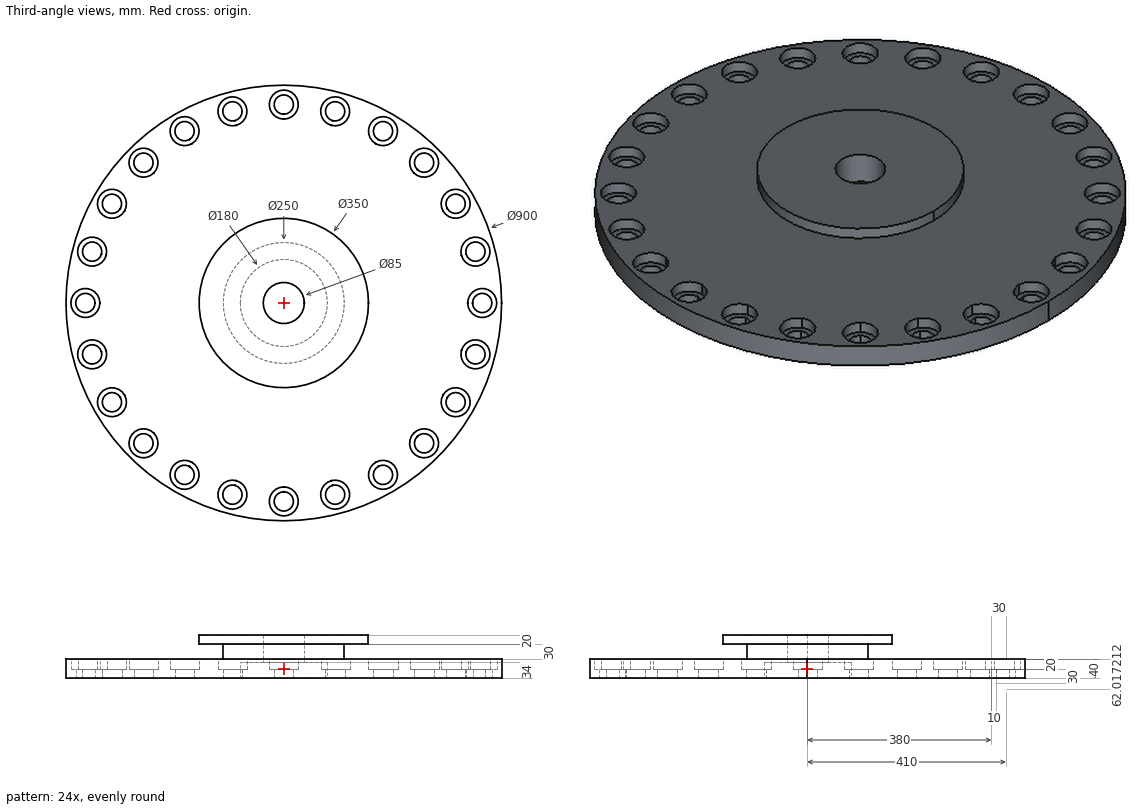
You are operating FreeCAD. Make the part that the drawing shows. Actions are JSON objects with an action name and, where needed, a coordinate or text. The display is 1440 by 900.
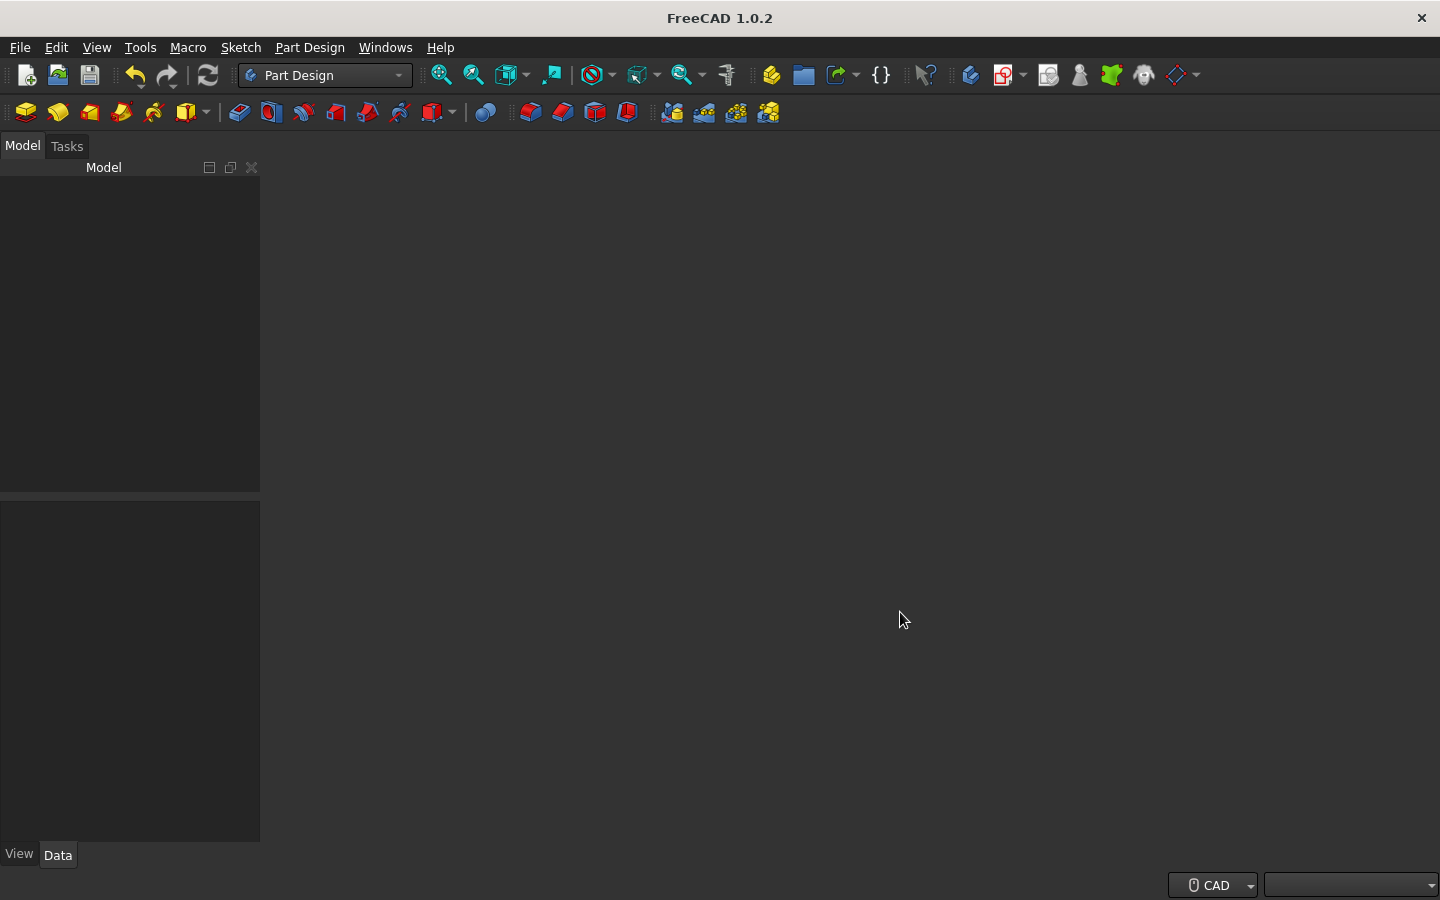
{"action": "key", "text": "ctrl+n"}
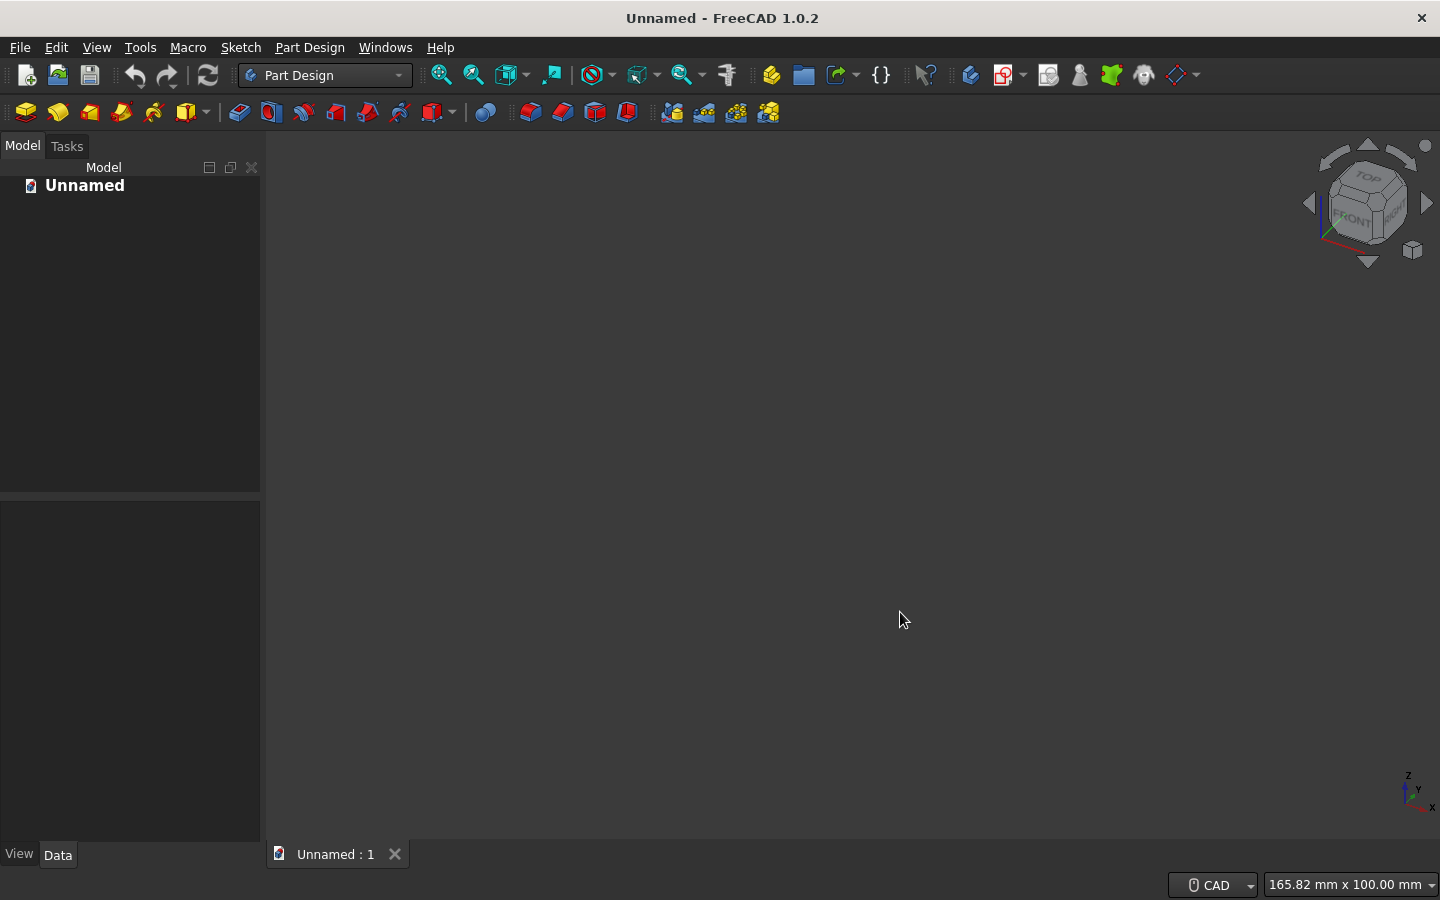
{"action": "left_click", "coordinate": [1004, 76]}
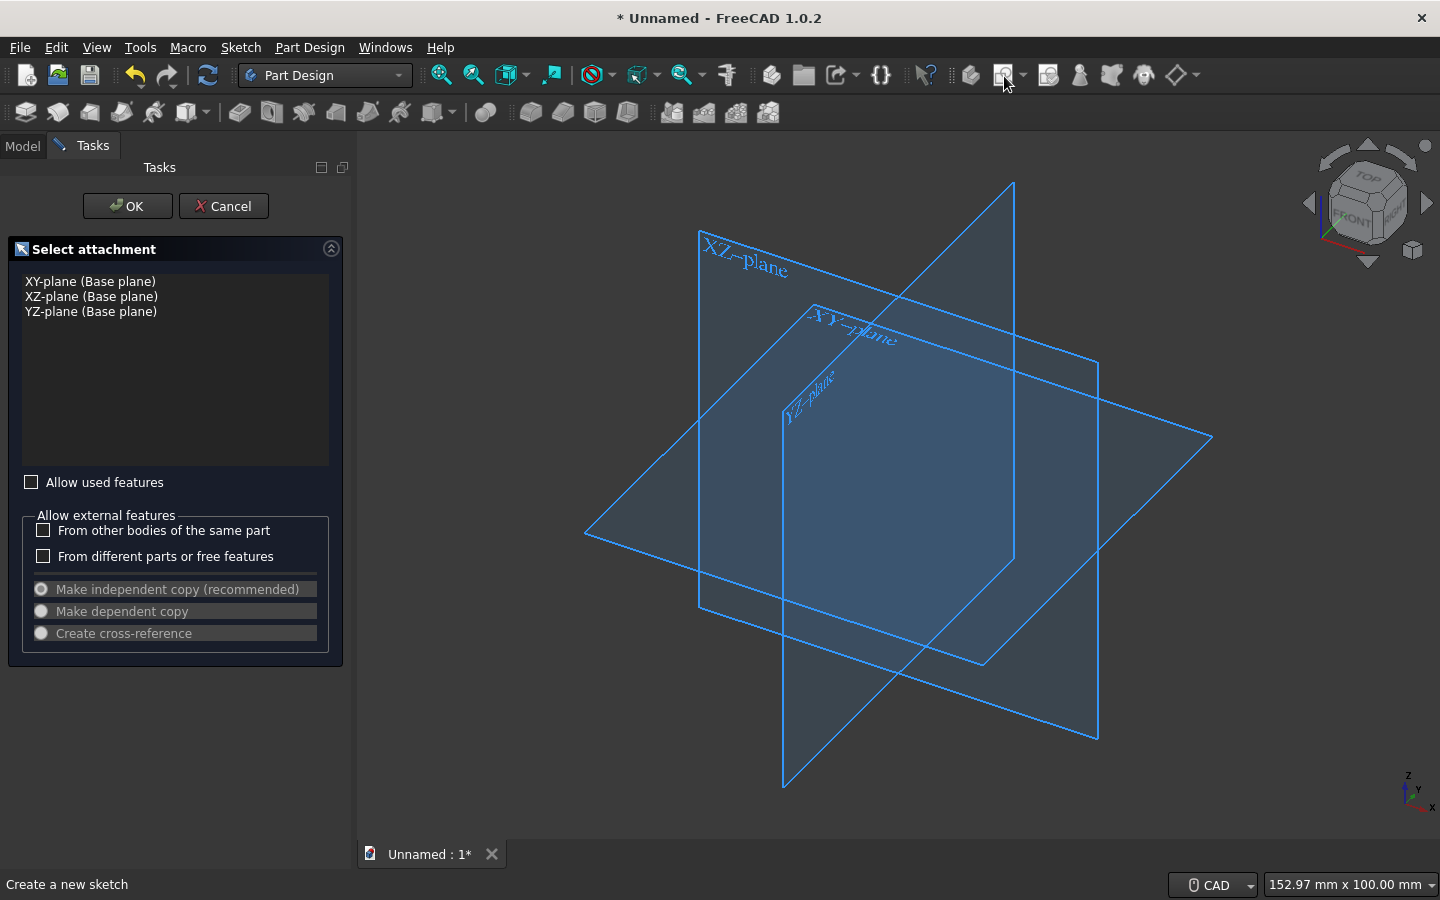
{"action": "left_click", "coordinate": [82, 282]}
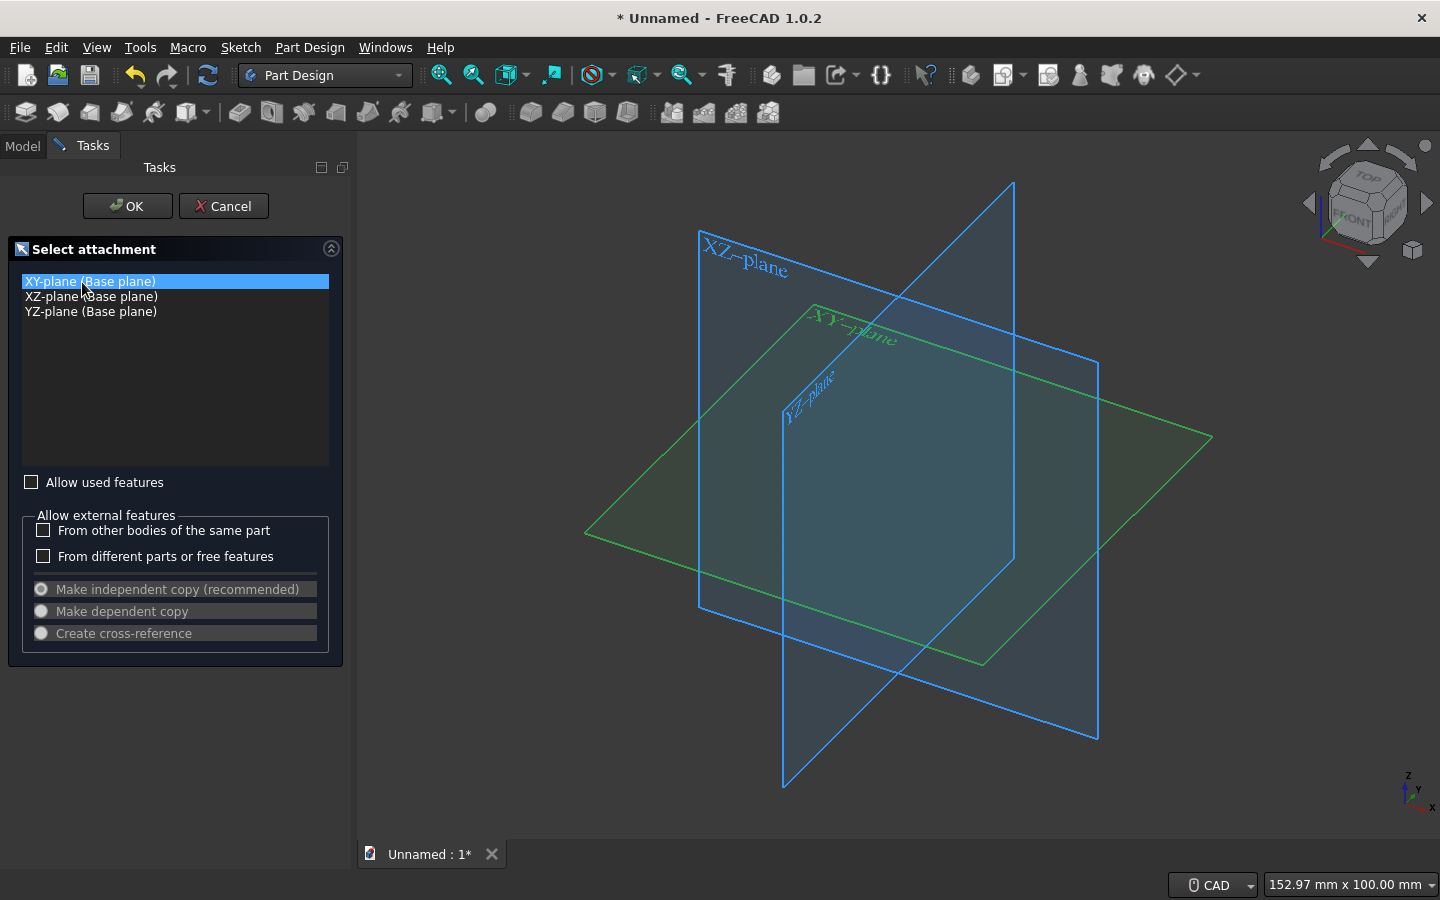
{"action": "left_click", "coordinate": [128, 206]}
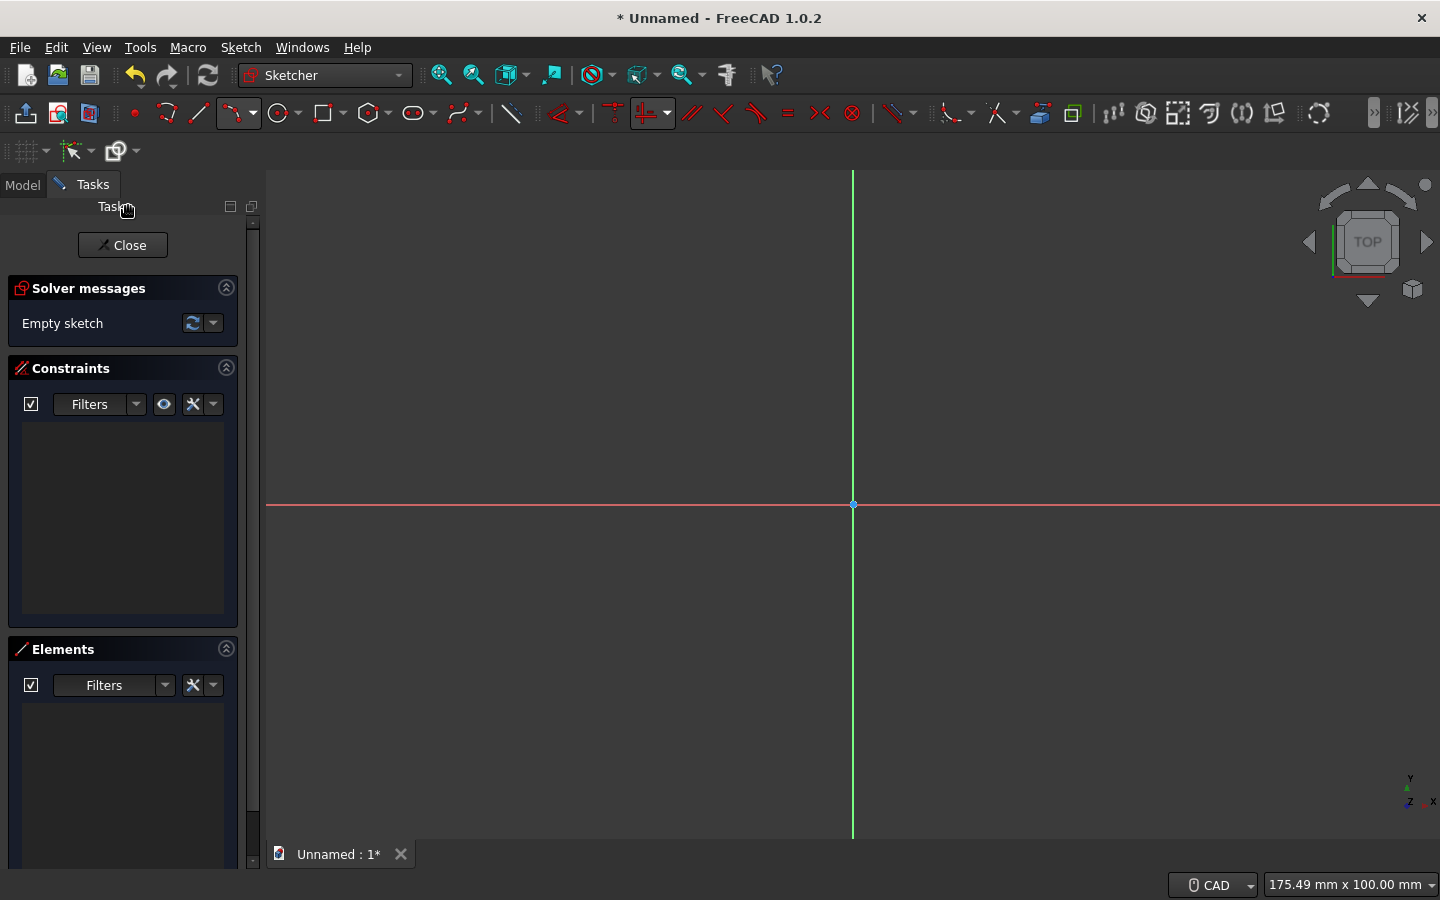
{"action": "scroll", "coordinate": [779, 504], "scroll_direction": "down", "scroll_amount": 13}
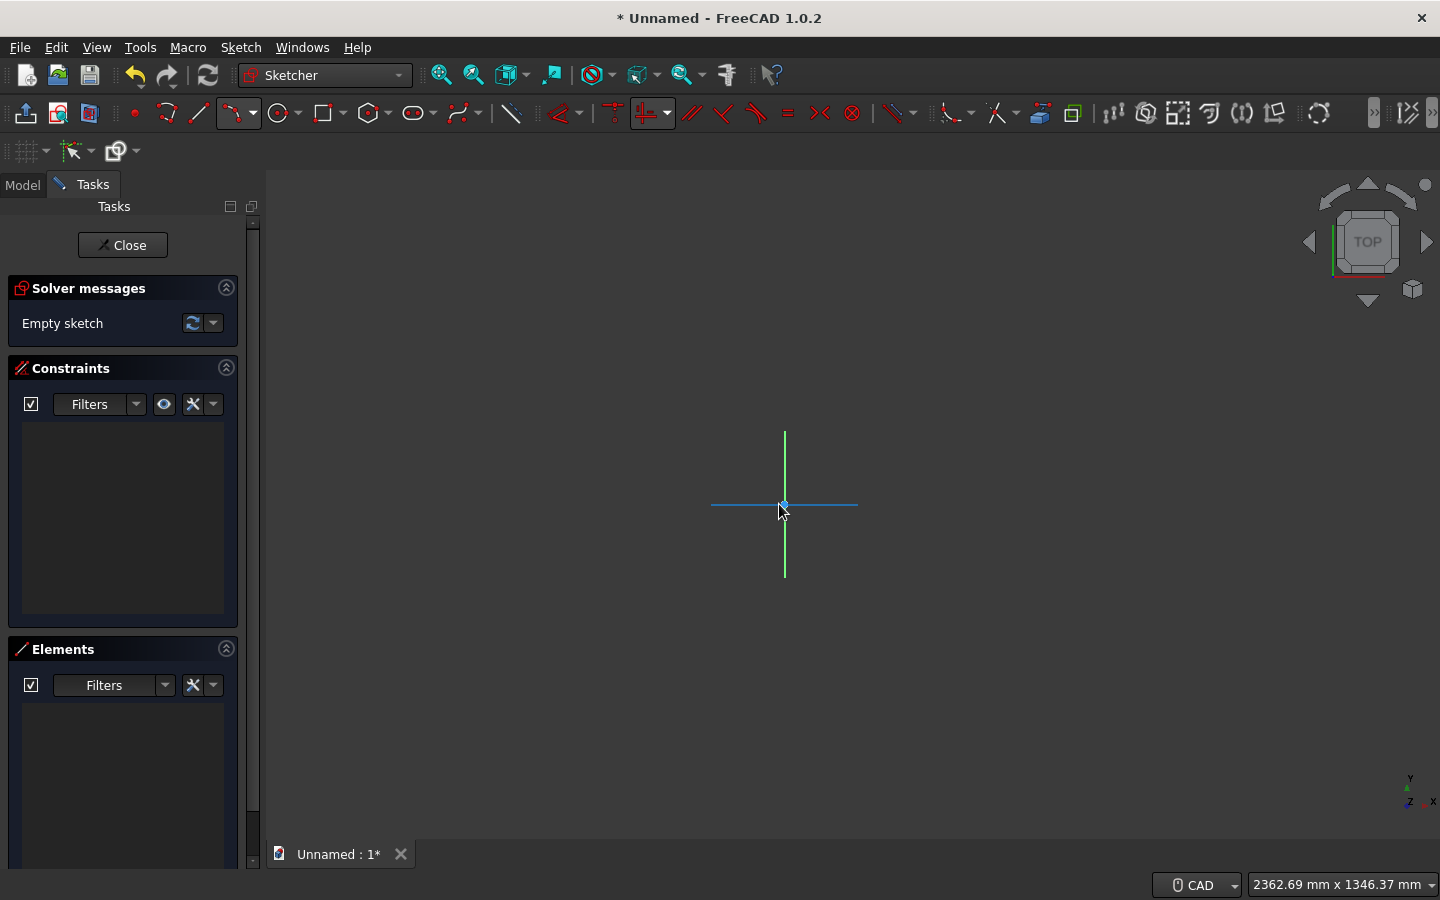
{"action": "key", "text": "g c"}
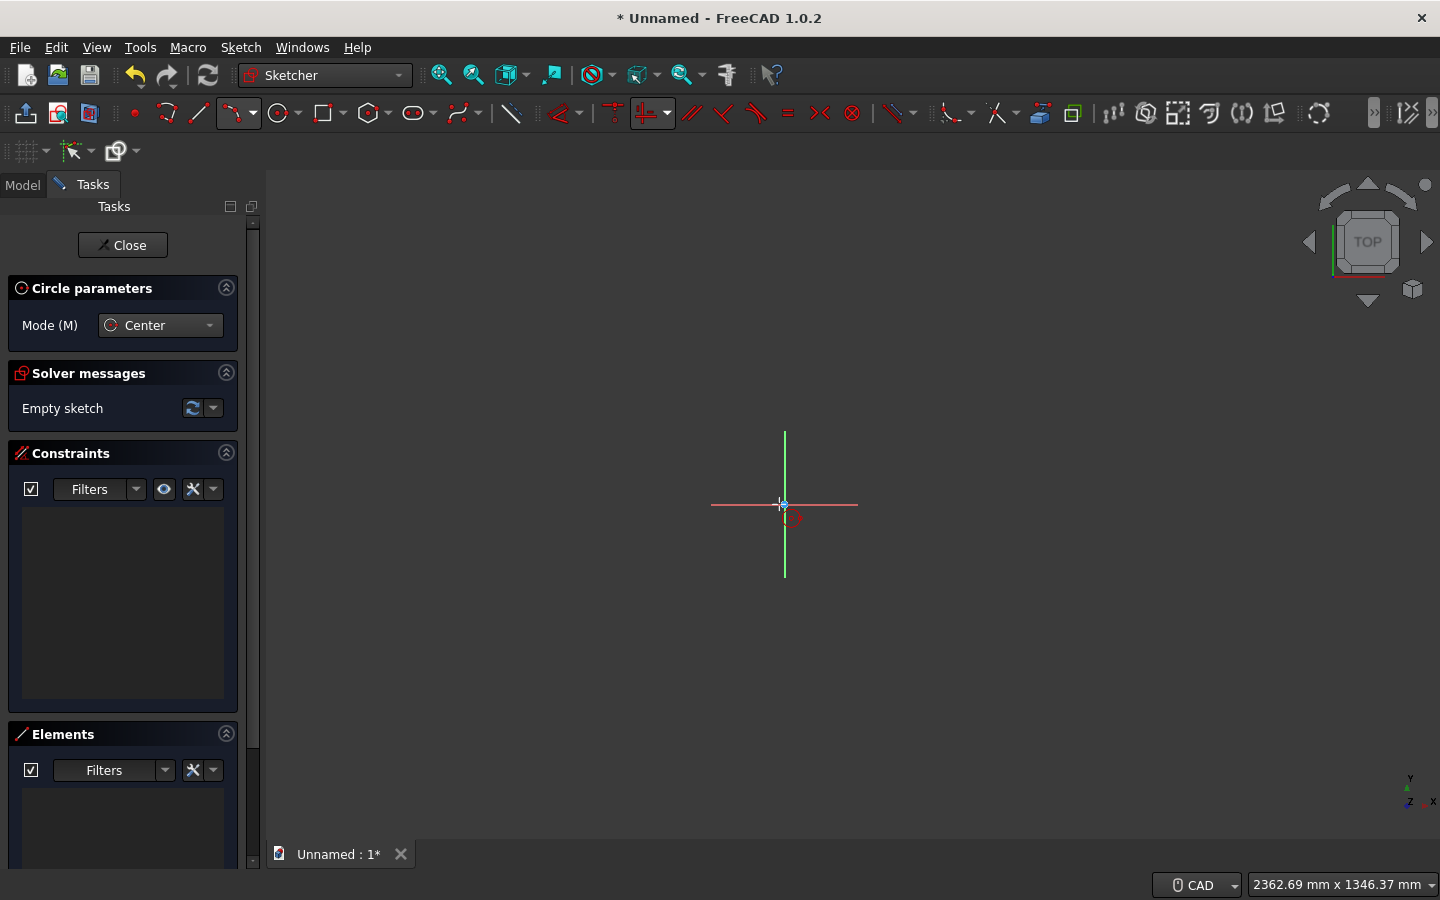
{"action": "left_click", "coordinate": [785, 504]}
{"action": "mouse_move", "coordinate": [943, 346]}